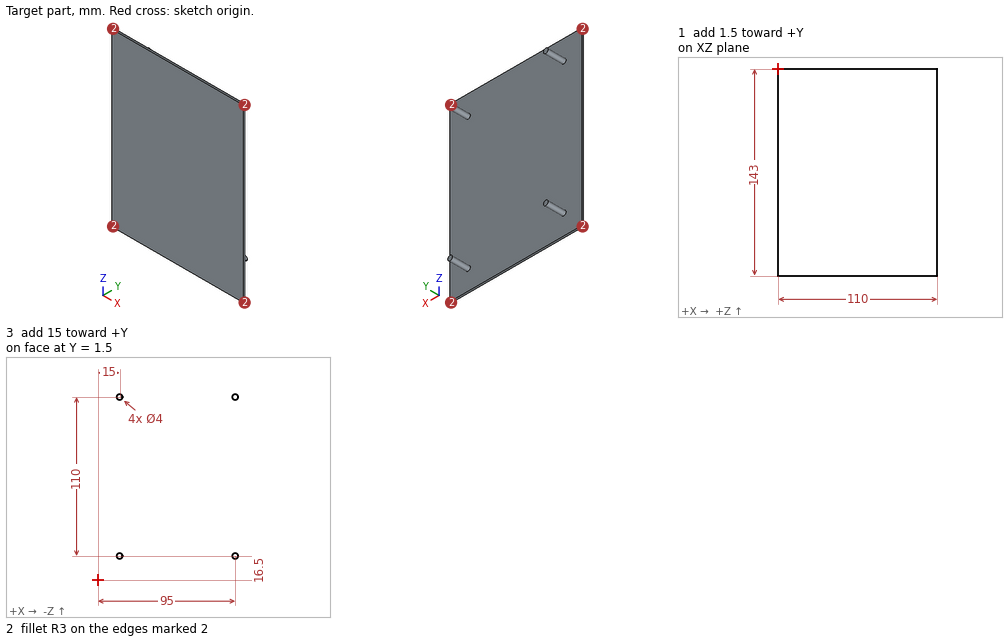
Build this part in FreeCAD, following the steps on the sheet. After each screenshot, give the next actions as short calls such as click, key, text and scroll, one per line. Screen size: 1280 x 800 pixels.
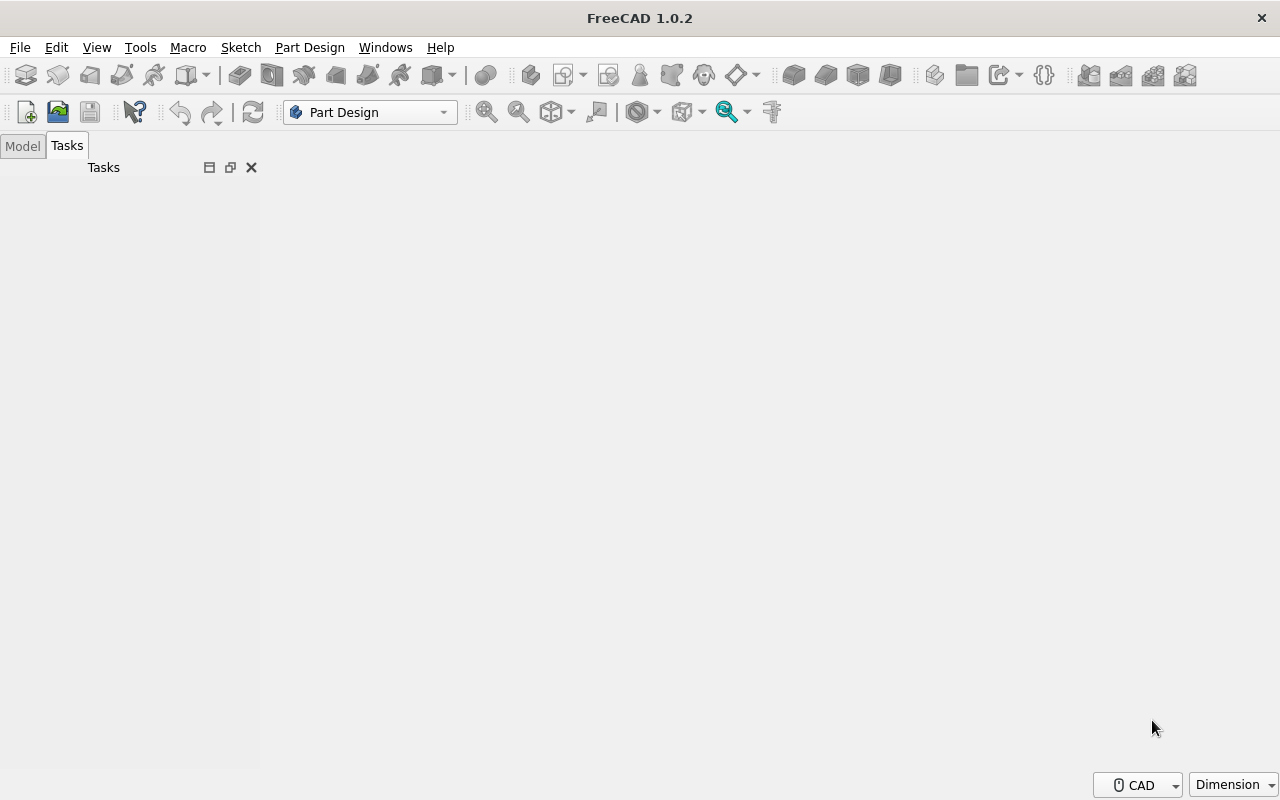
click(26, 112)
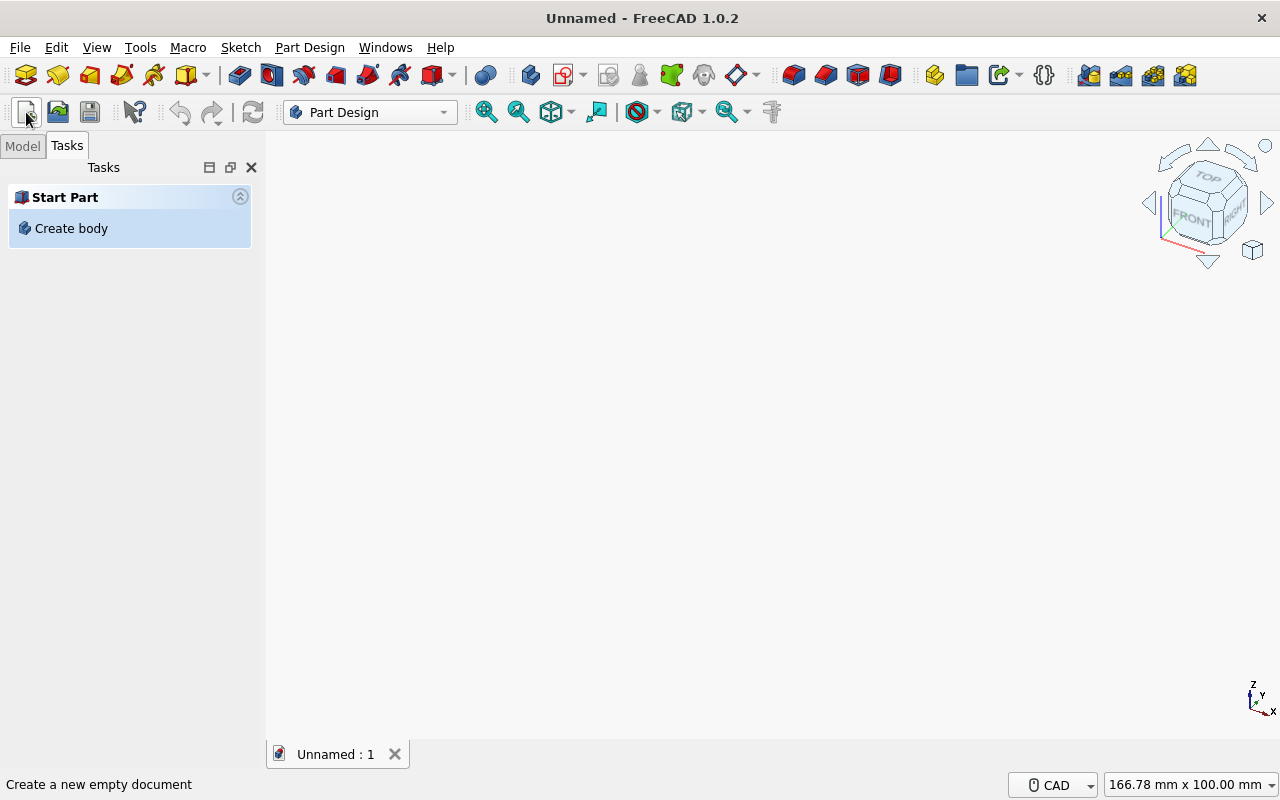
click(564, 76)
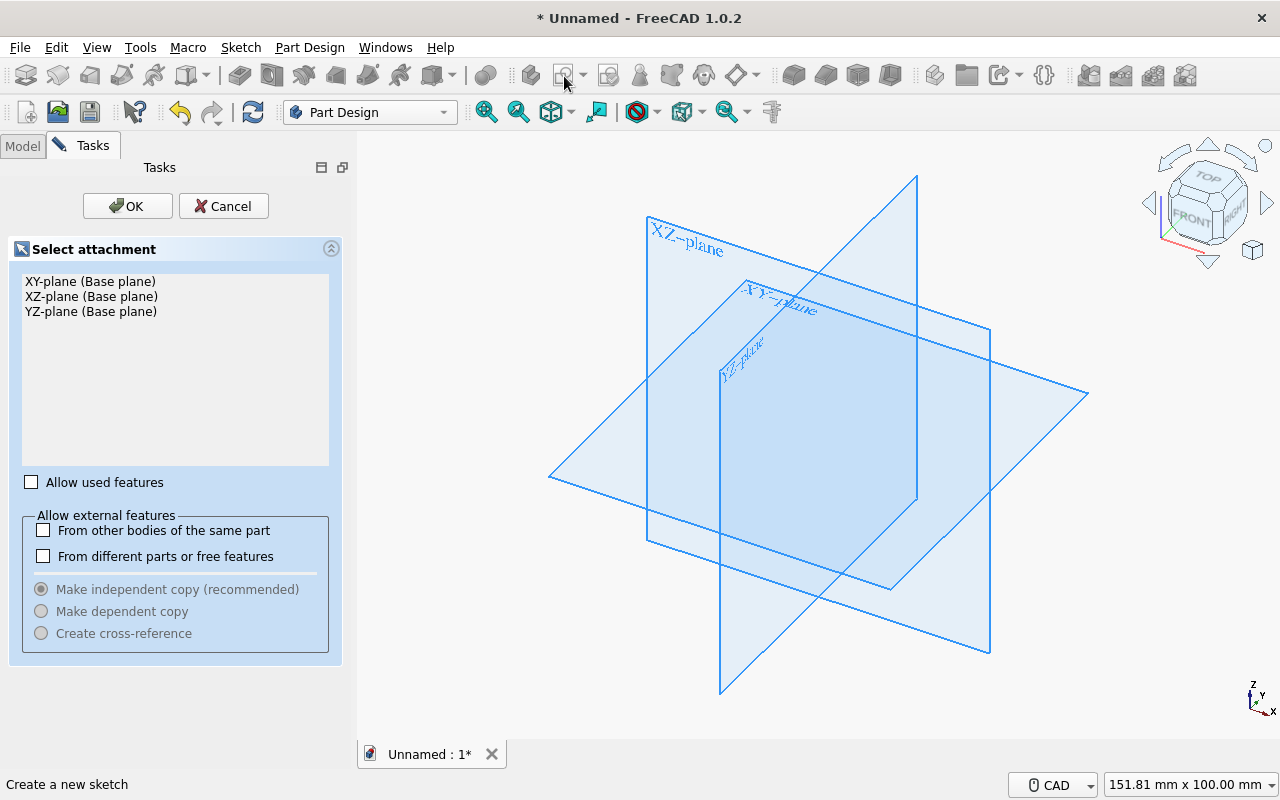
click(82, 296)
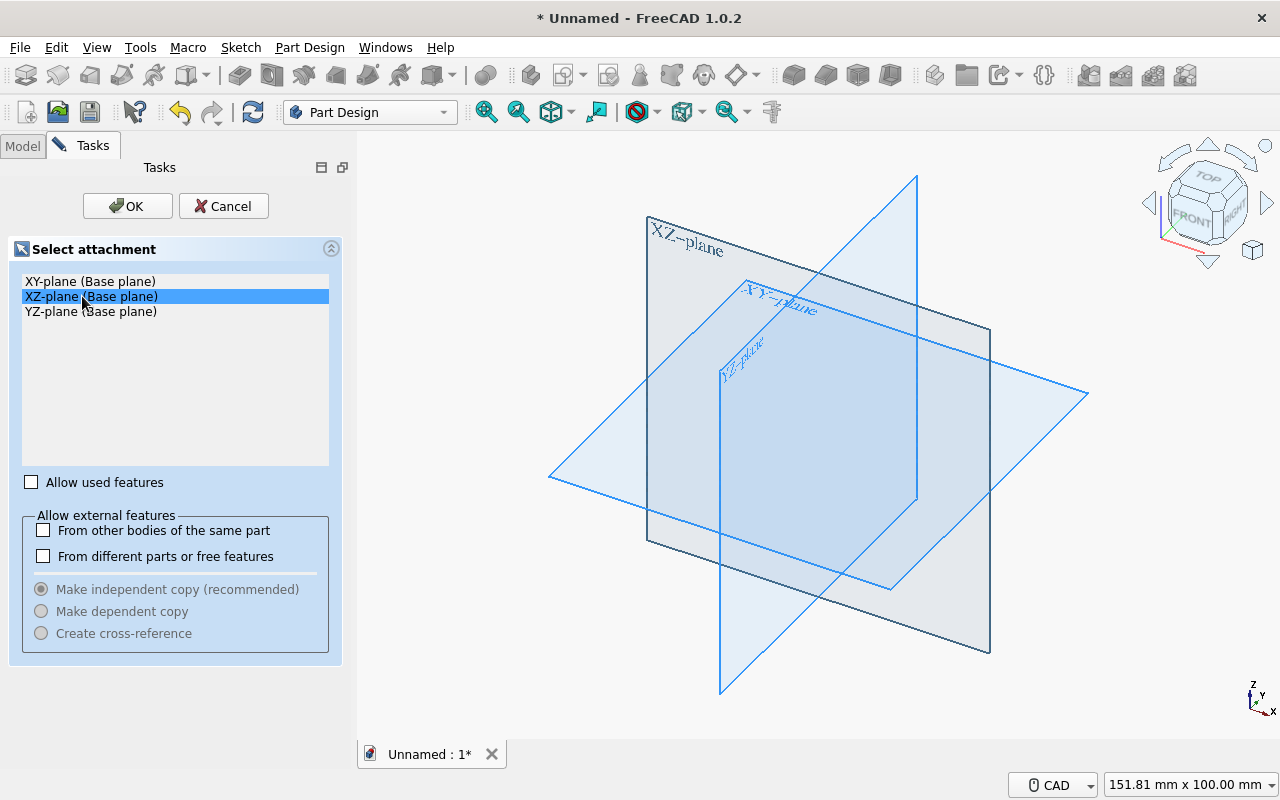
click(128, 206)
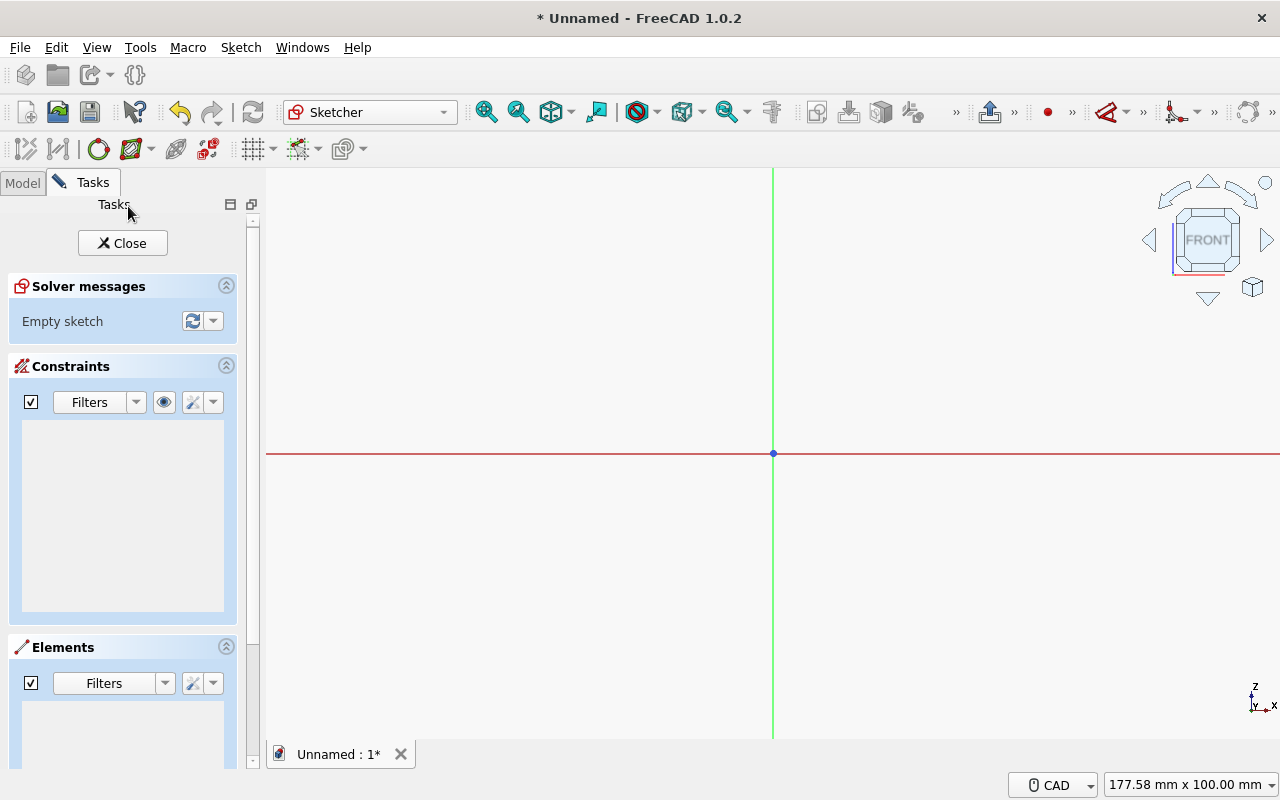
scroll(392, 196, down, 4)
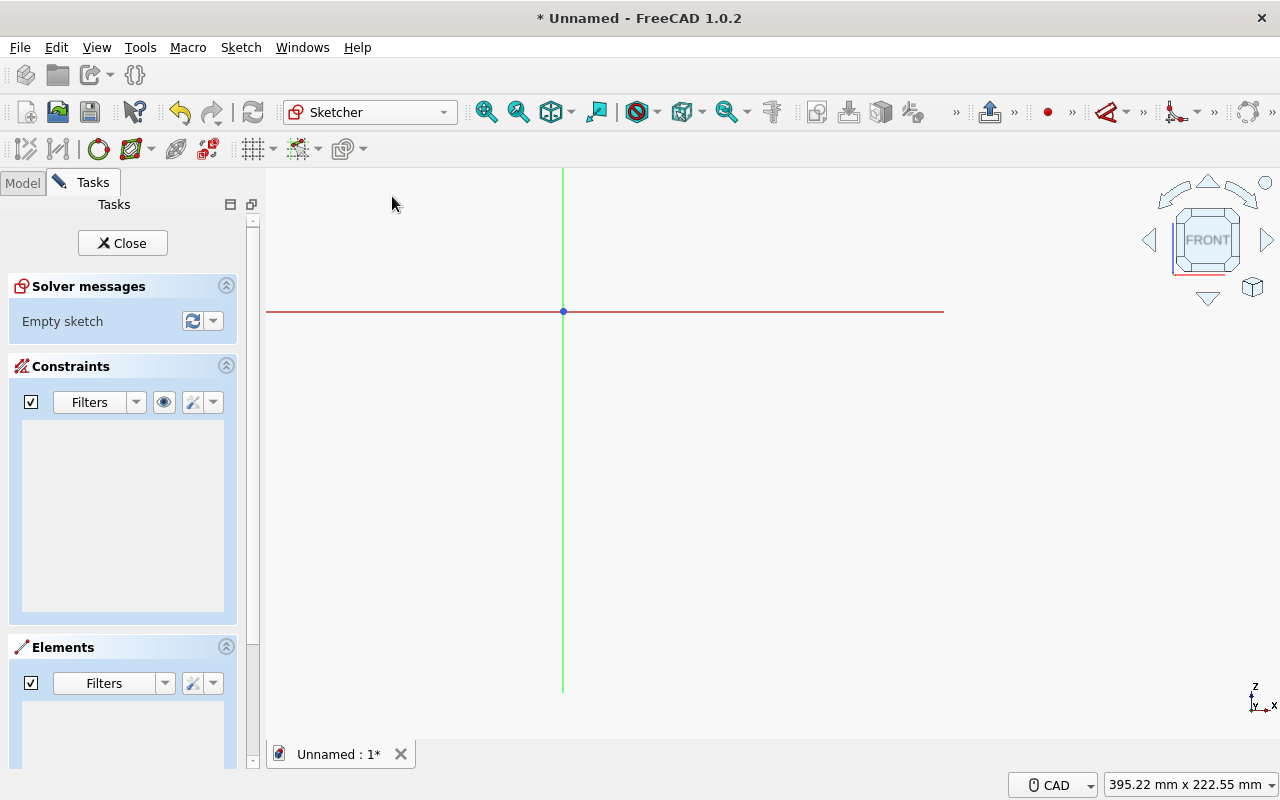
key(g)
key(r)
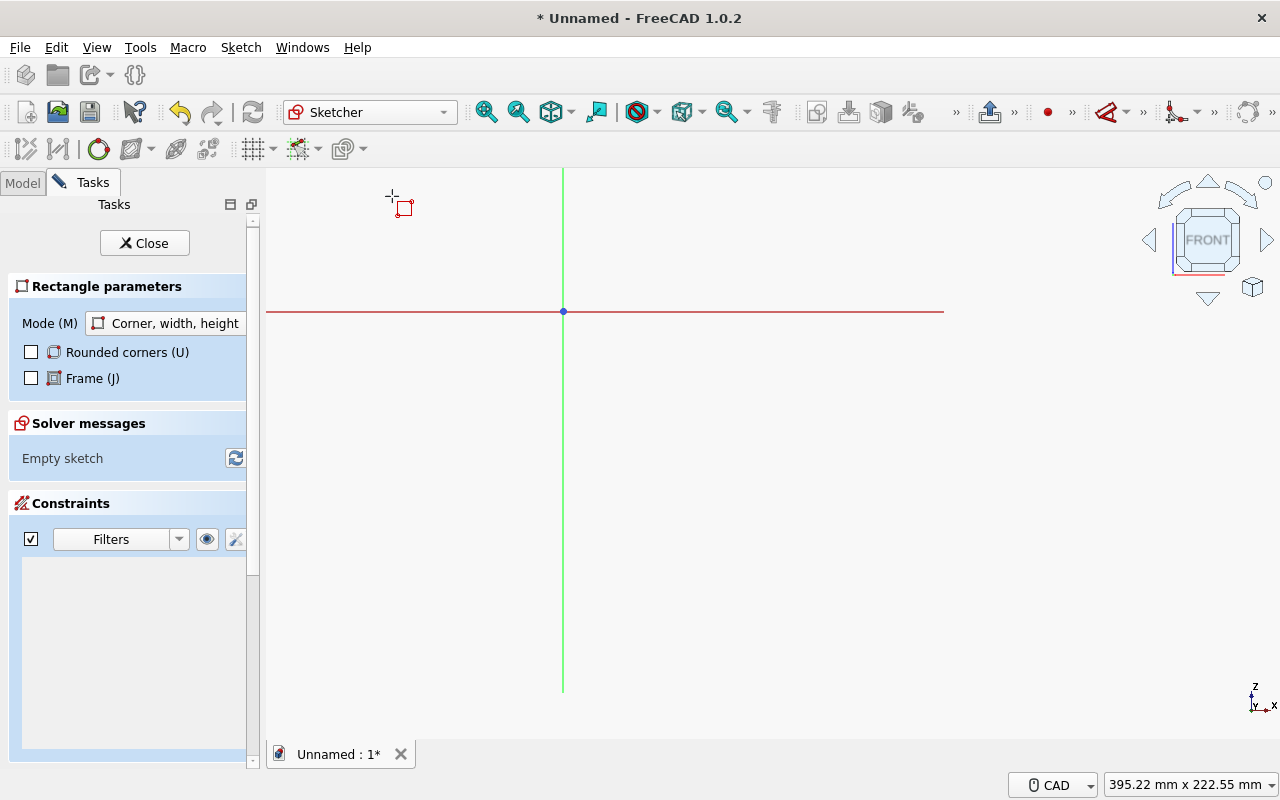
click(563, 312)
click(845, 679)
key(Escape)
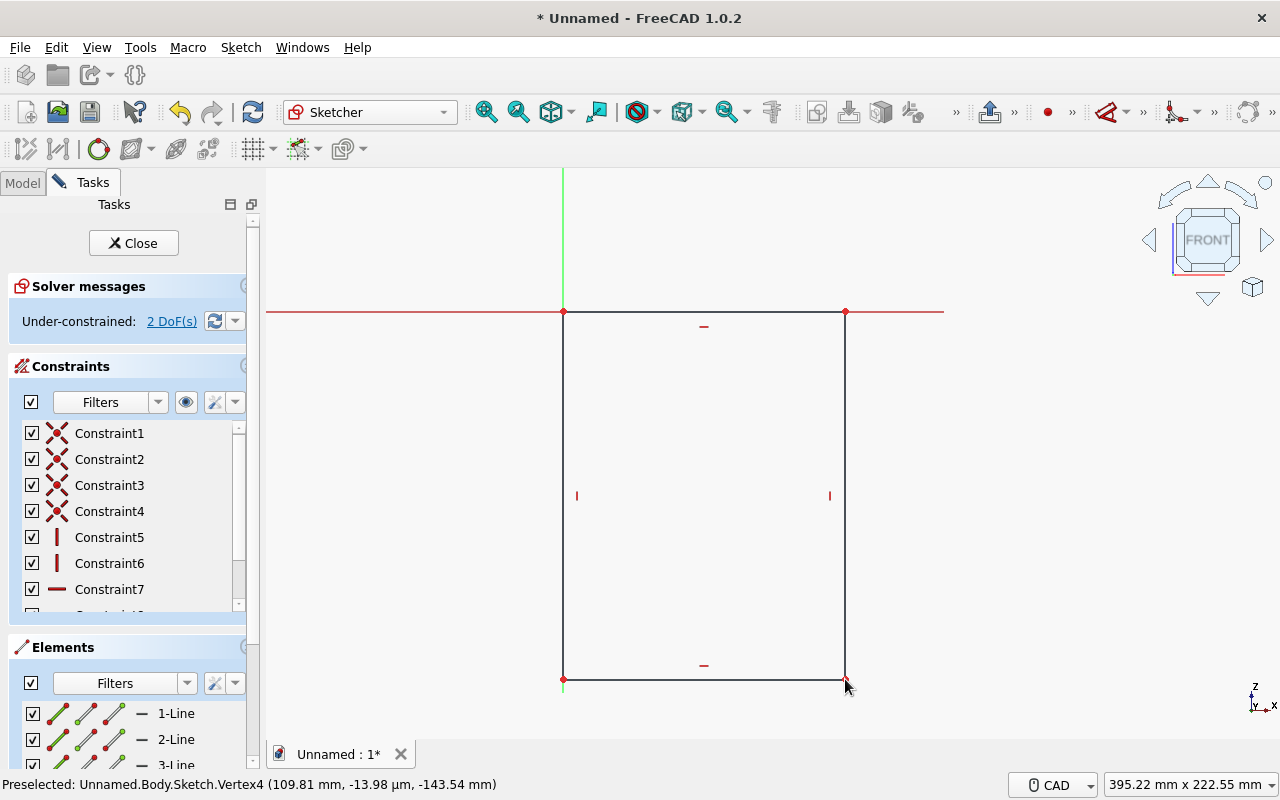
click(1106, 112)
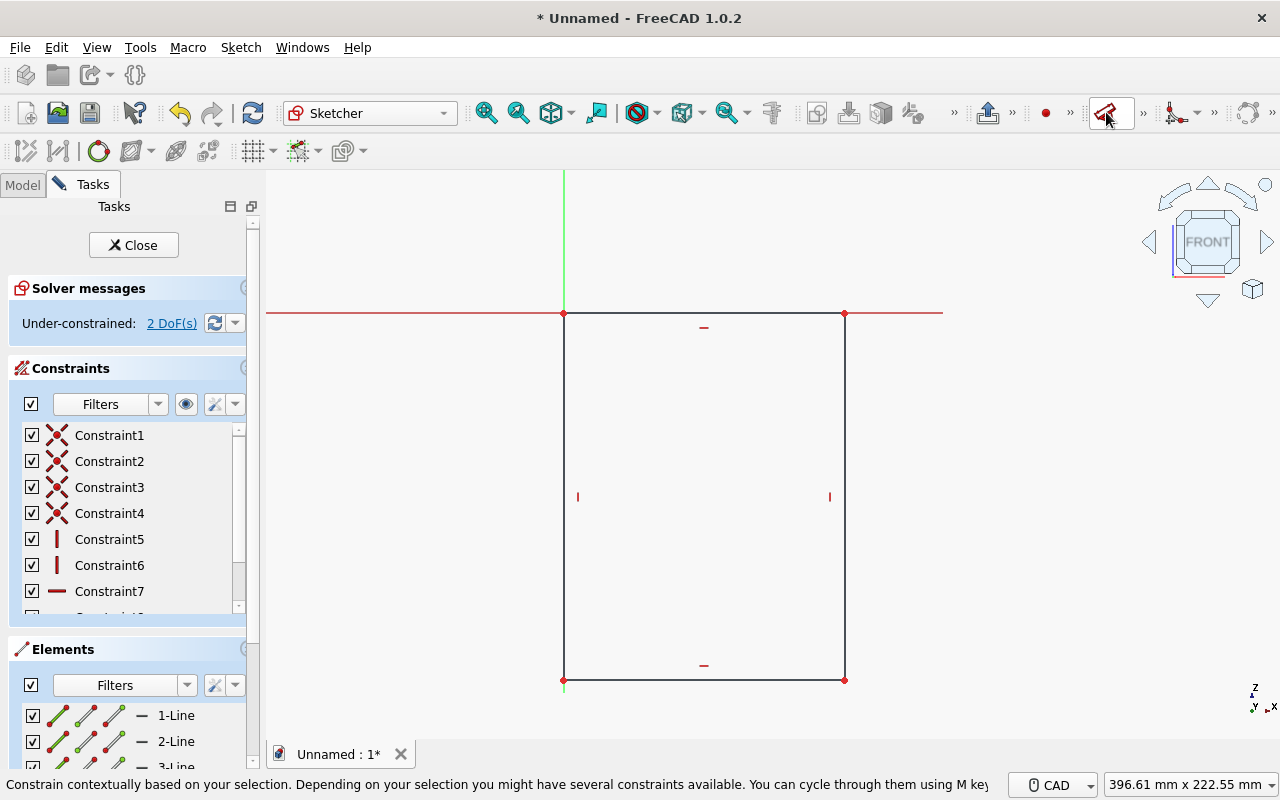
click(564, 423)
click(530, 497)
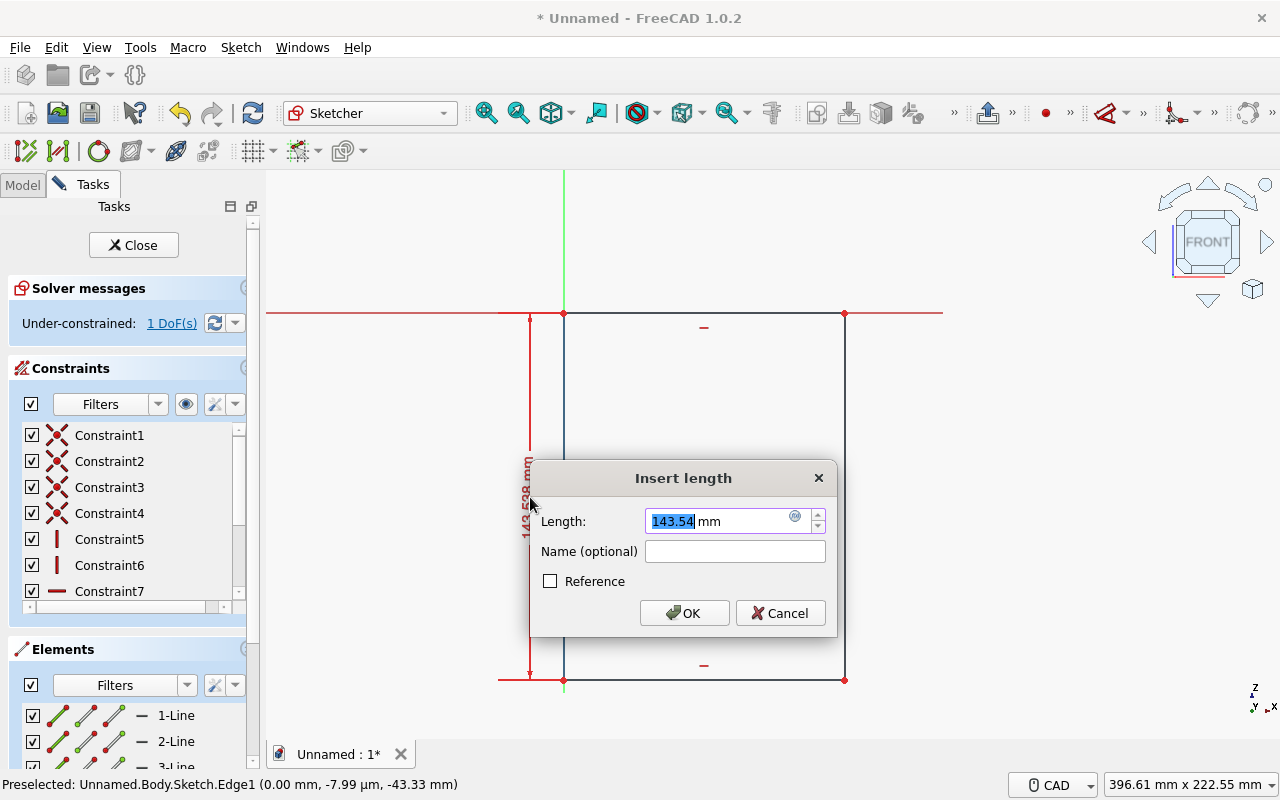
text(143)
key(Return)